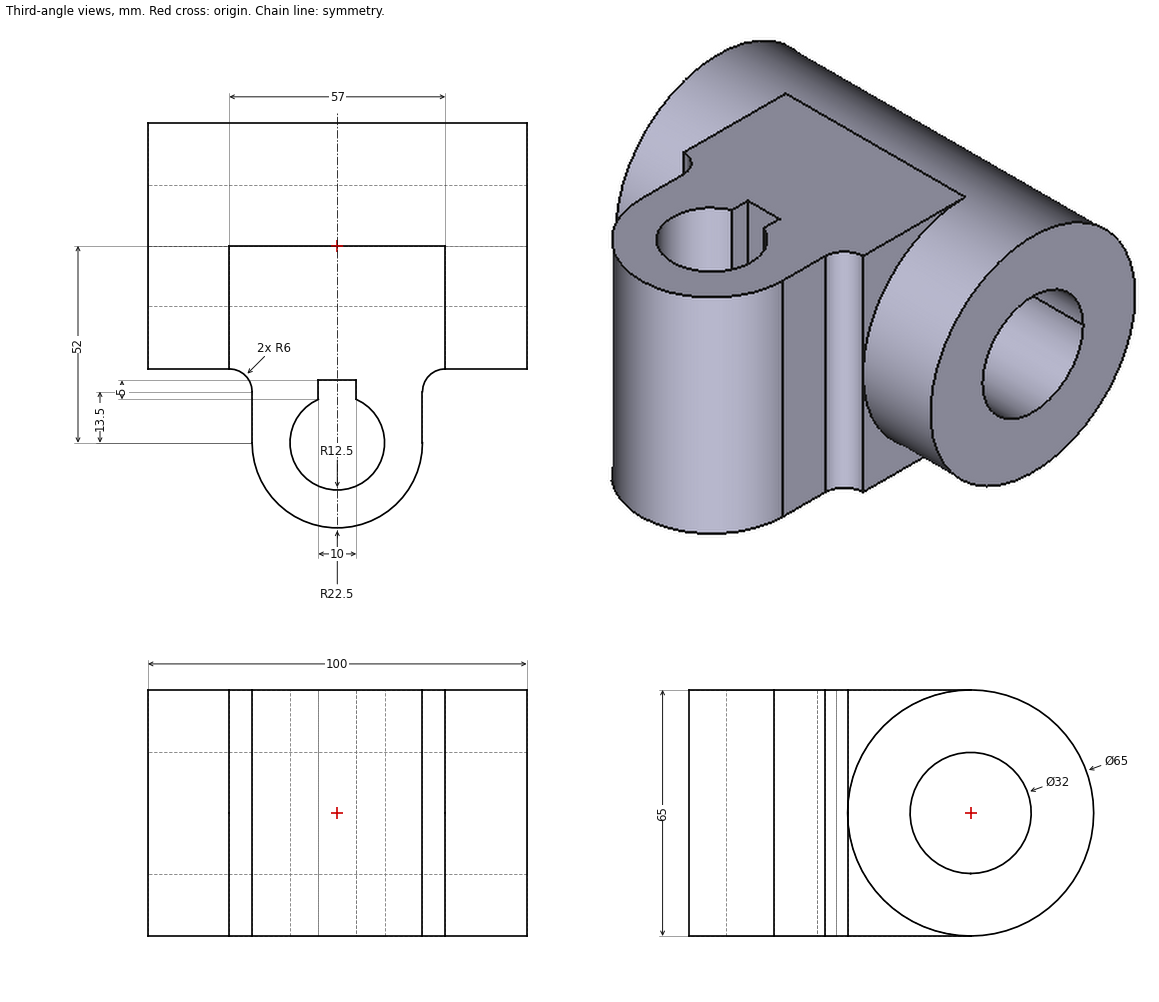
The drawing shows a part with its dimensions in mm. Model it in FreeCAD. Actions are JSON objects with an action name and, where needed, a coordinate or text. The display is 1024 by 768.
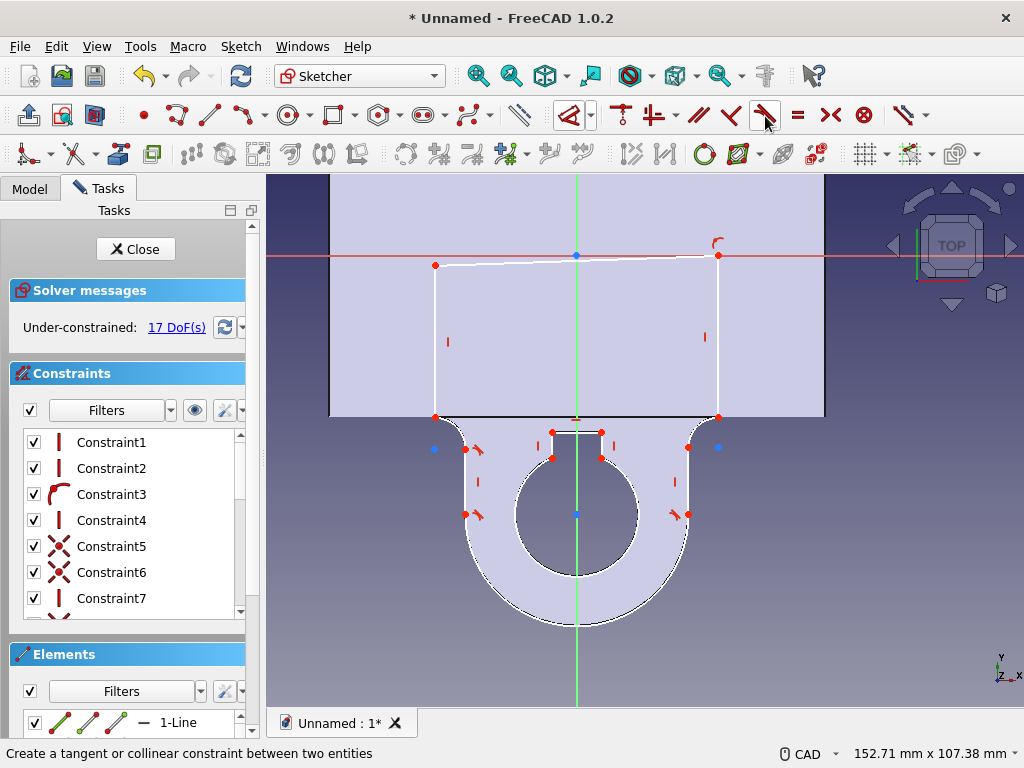
{"action": "left_click", "coordinate": [688, 495]}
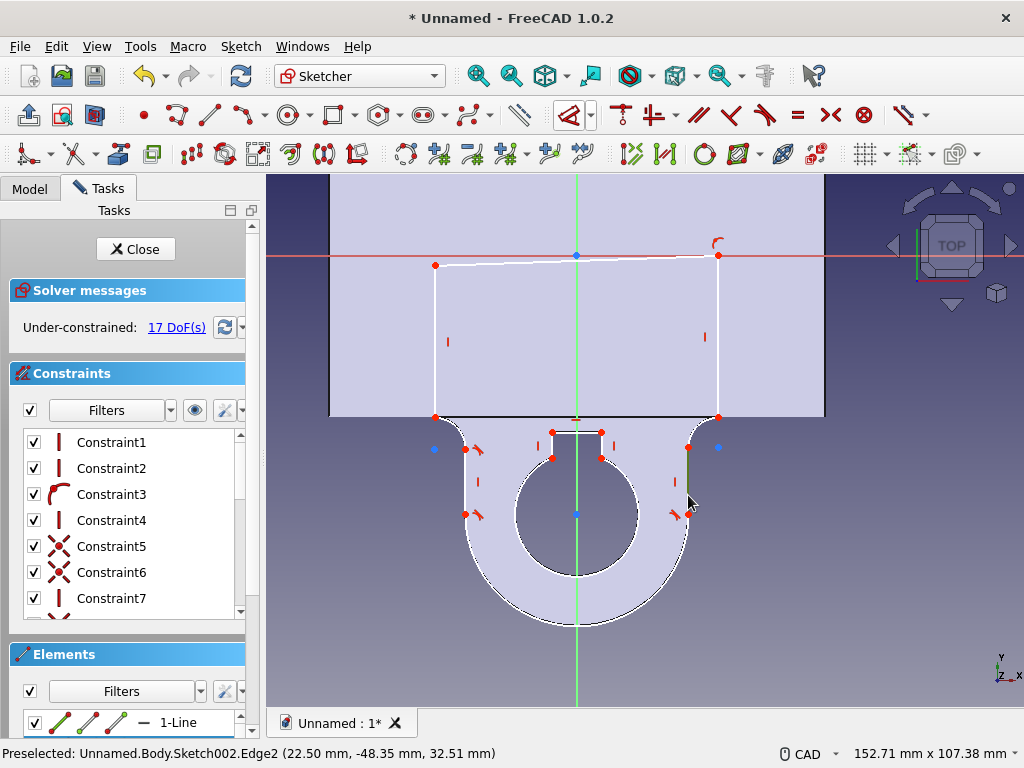
{"action": "left_click", "coordinate": [705, 421]}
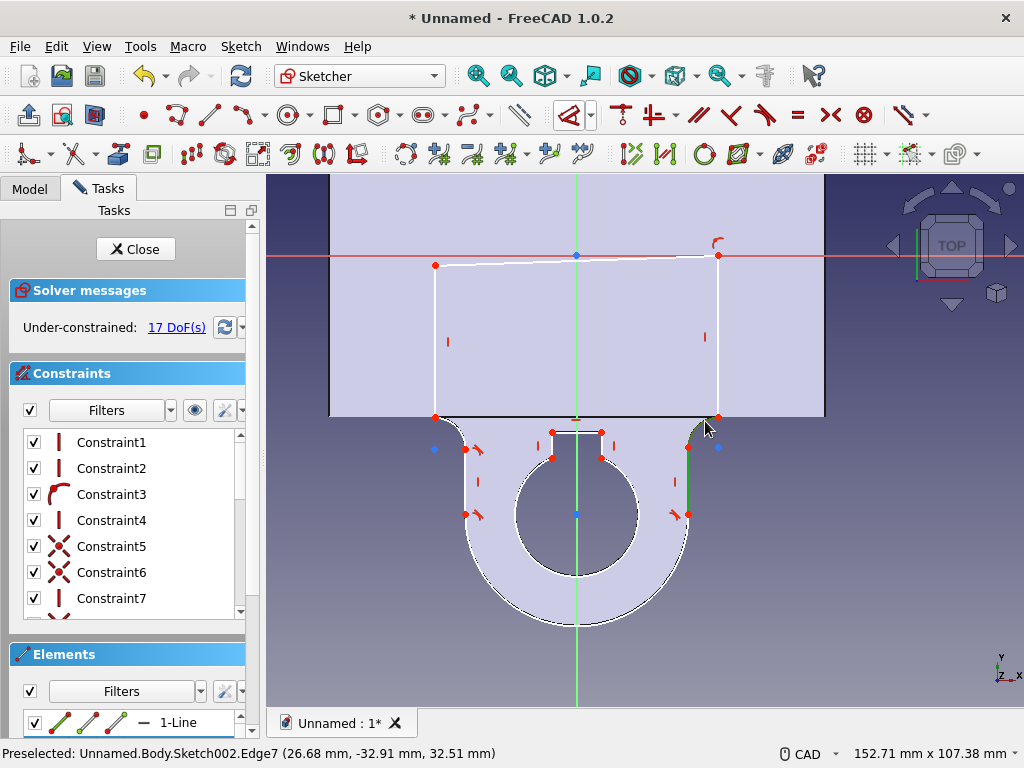
{"action": "key", "text": "t"}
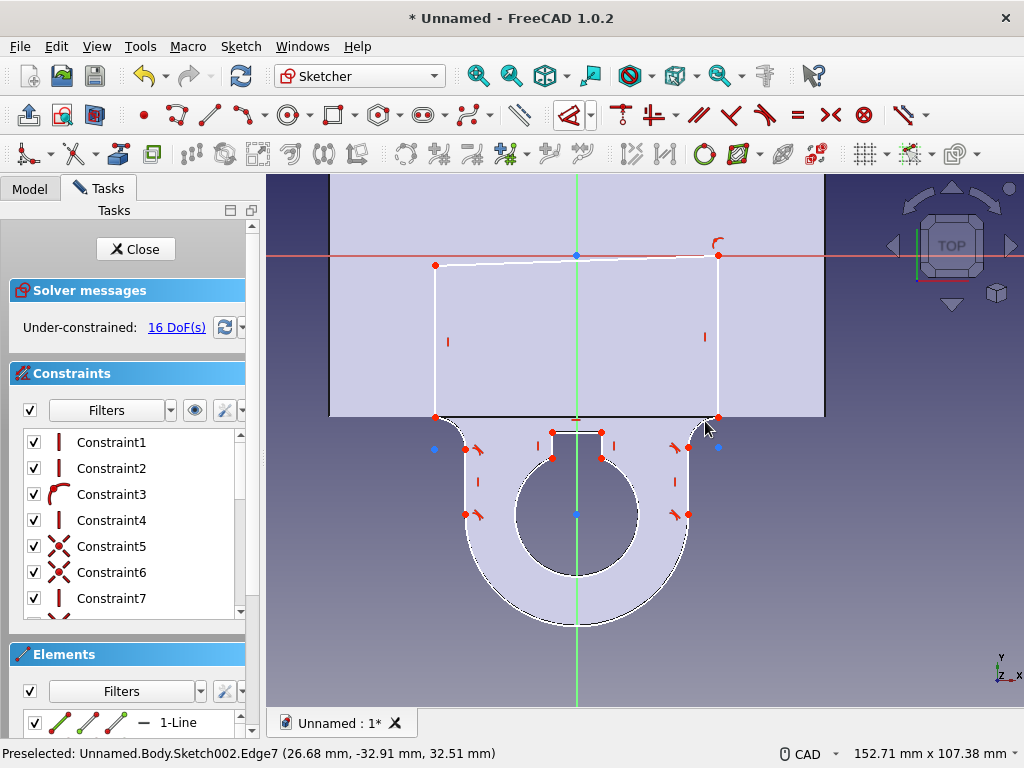
{"action": "left_click", "coordinate": [634, 259]}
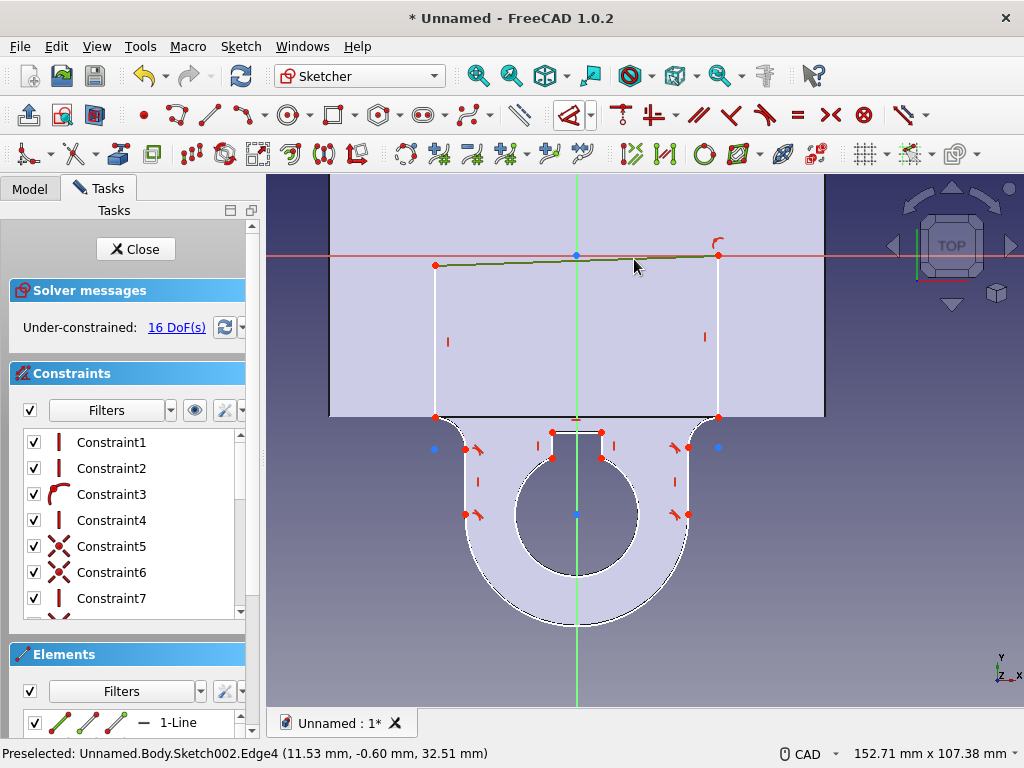
{"action": "left_click", "coordinate": [676, 116]}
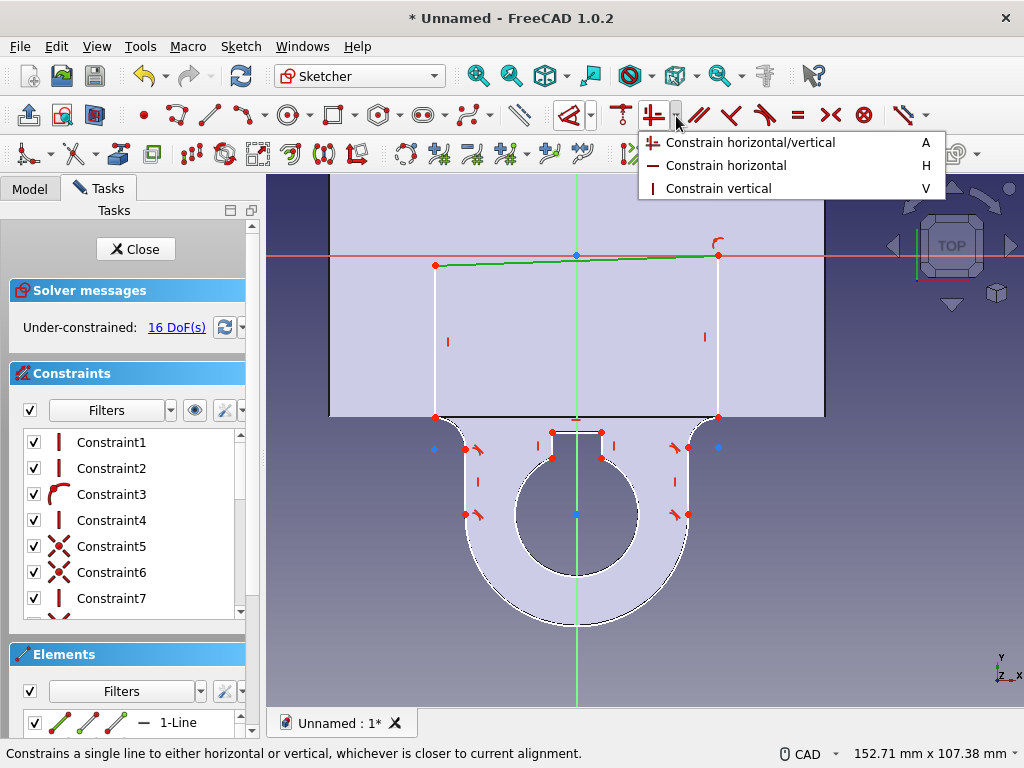
{"action": "left_click", "coordinate": [792, 166]}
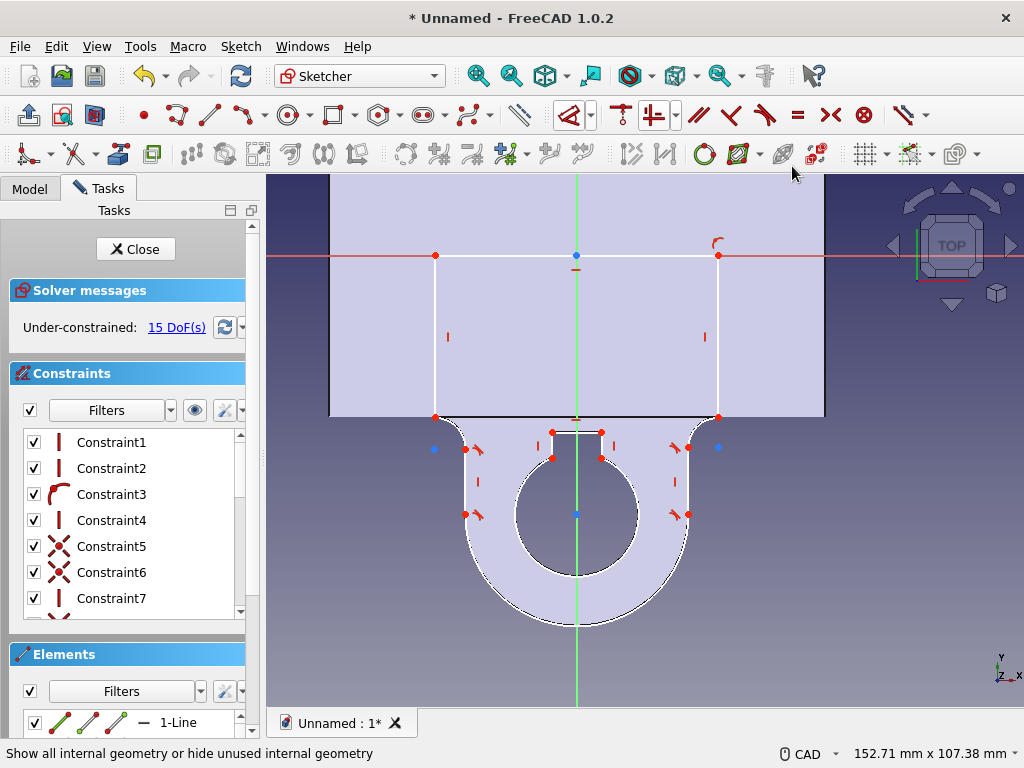
{"action": "left_click", "coordinate": [511, 605]}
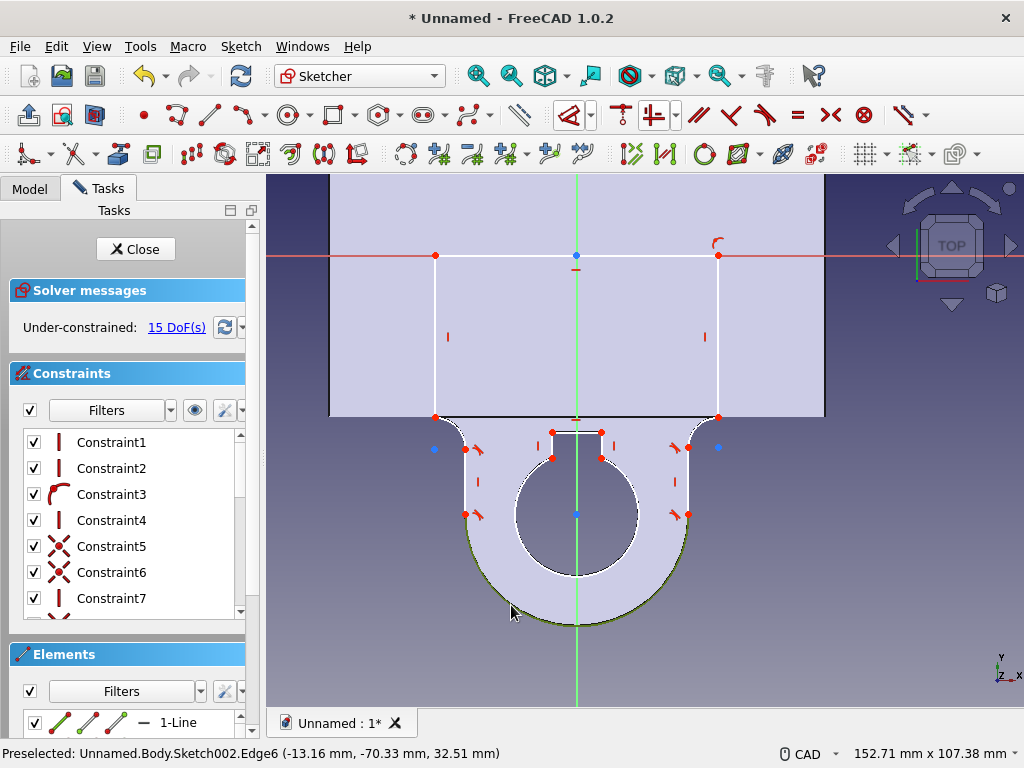
{"action": "left_click", "coordinate": [522, 543]}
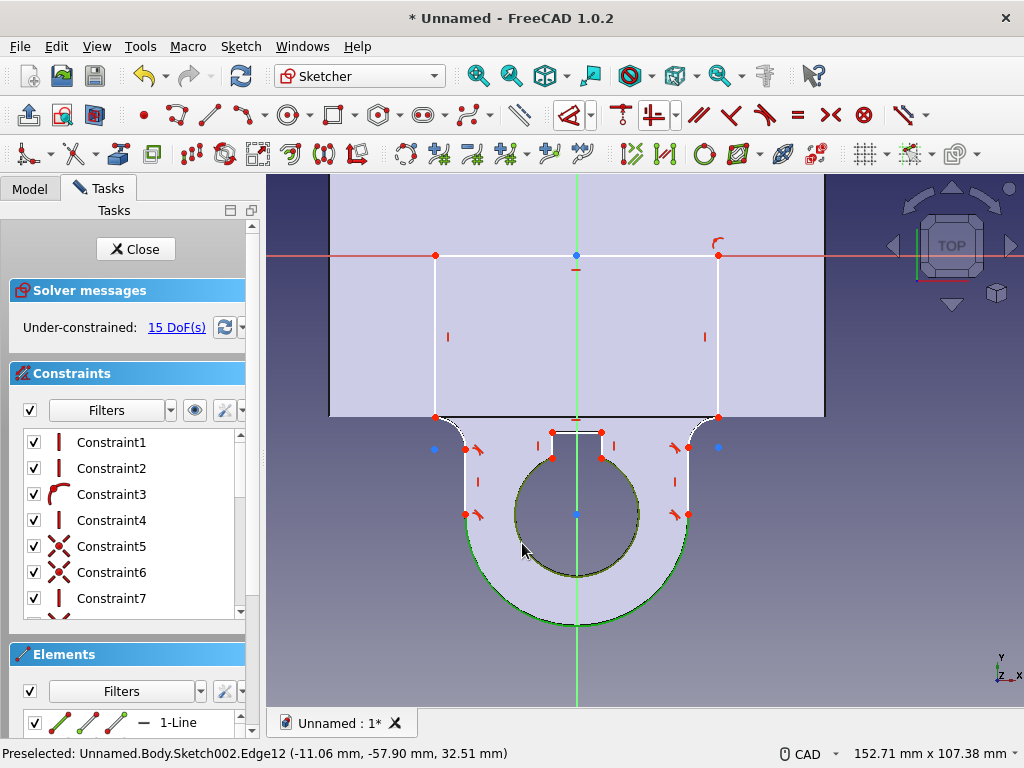
{"action": "key", "text": "c"}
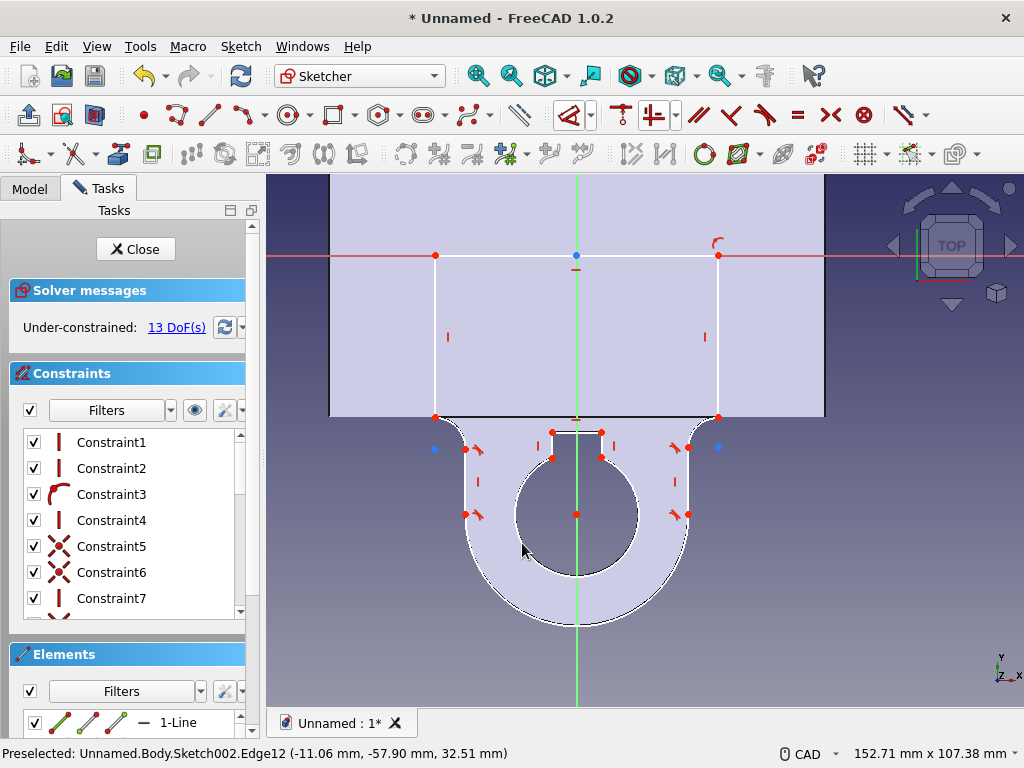
{"action": "left_click", "coordinate": [705, 421]}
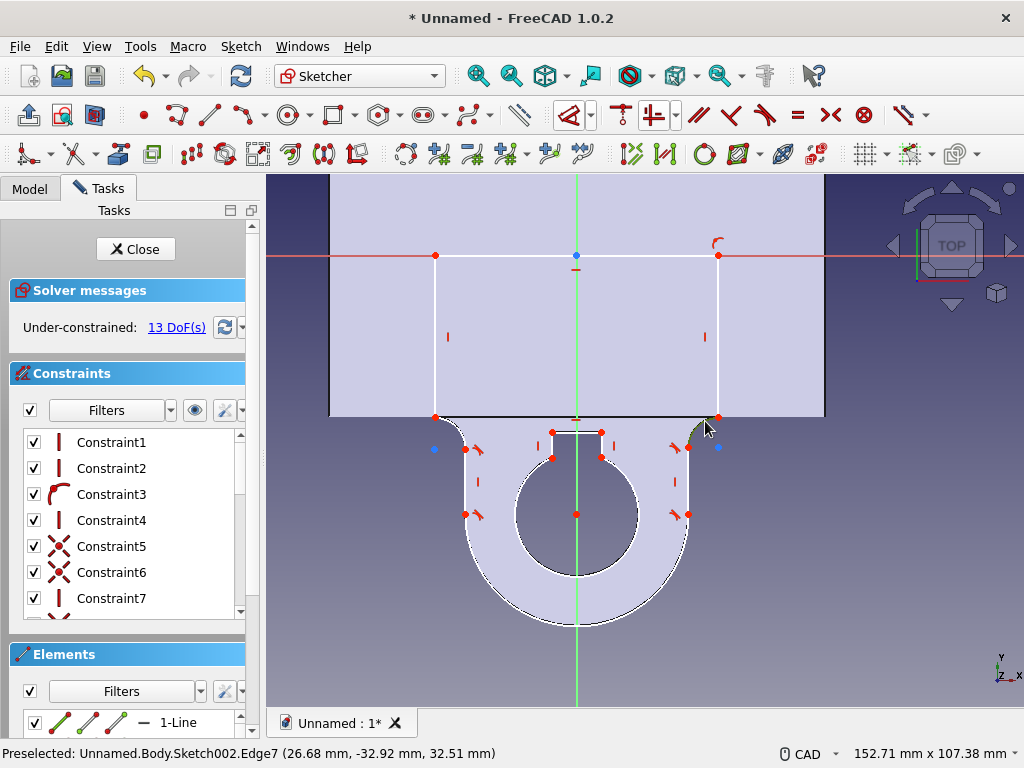
{"action": "left_click", "coordinate": [462, 435]}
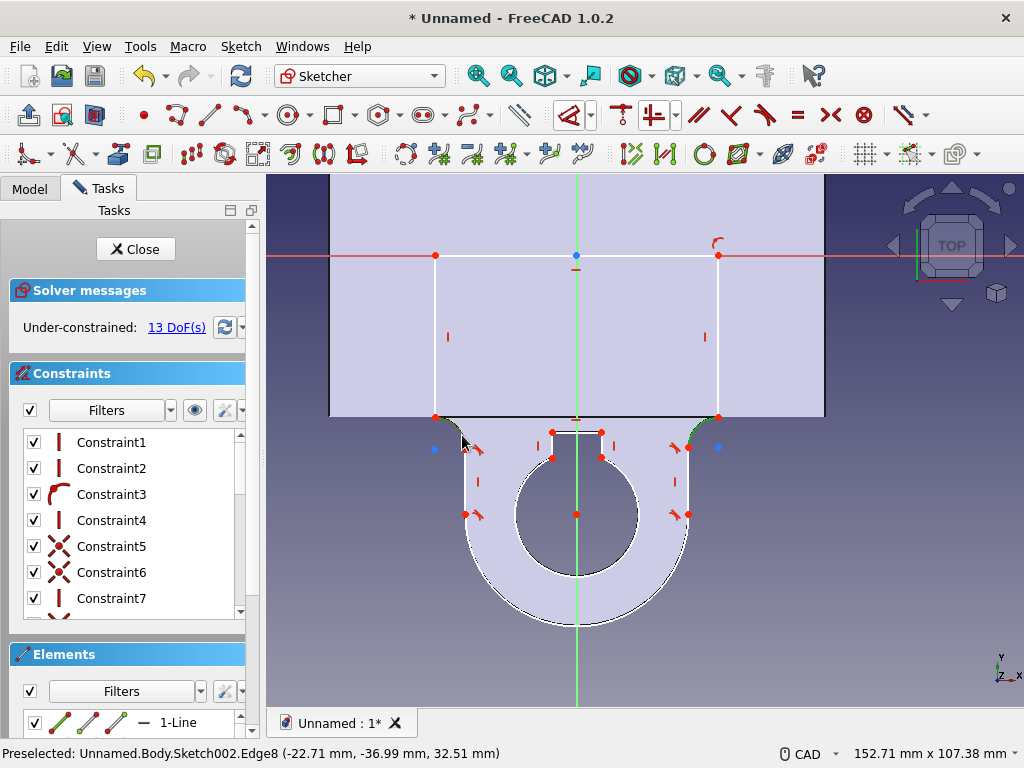
{"action": "key", "text": "e"}